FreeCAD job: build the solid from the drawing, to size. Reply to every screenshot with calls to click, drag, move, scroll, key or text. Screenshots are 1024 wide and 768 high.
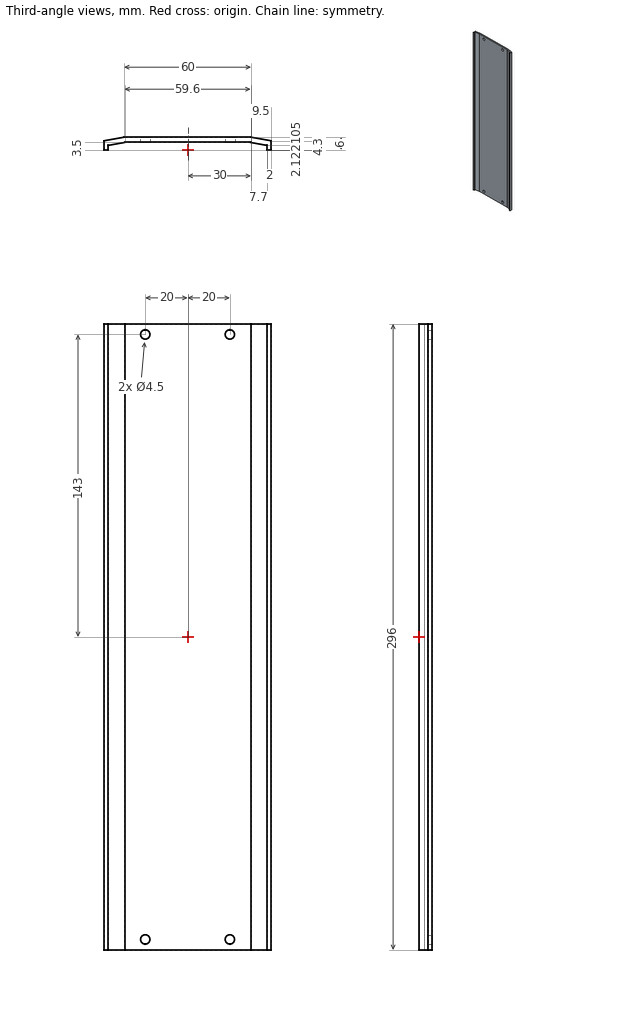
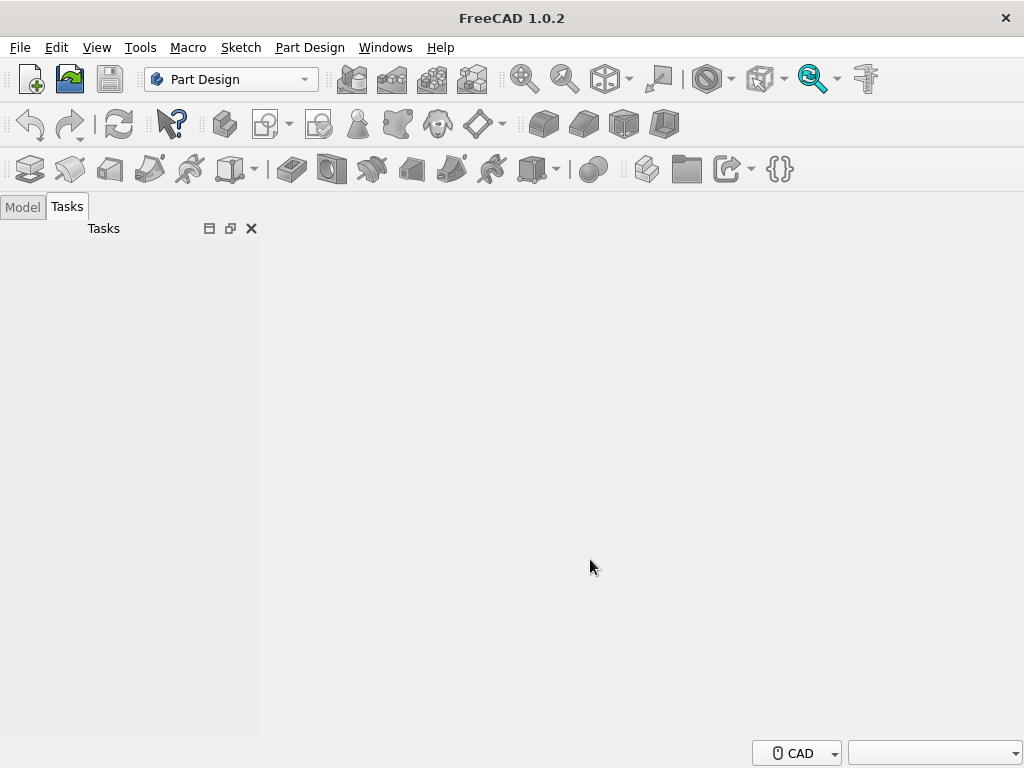
key(ctrl+n)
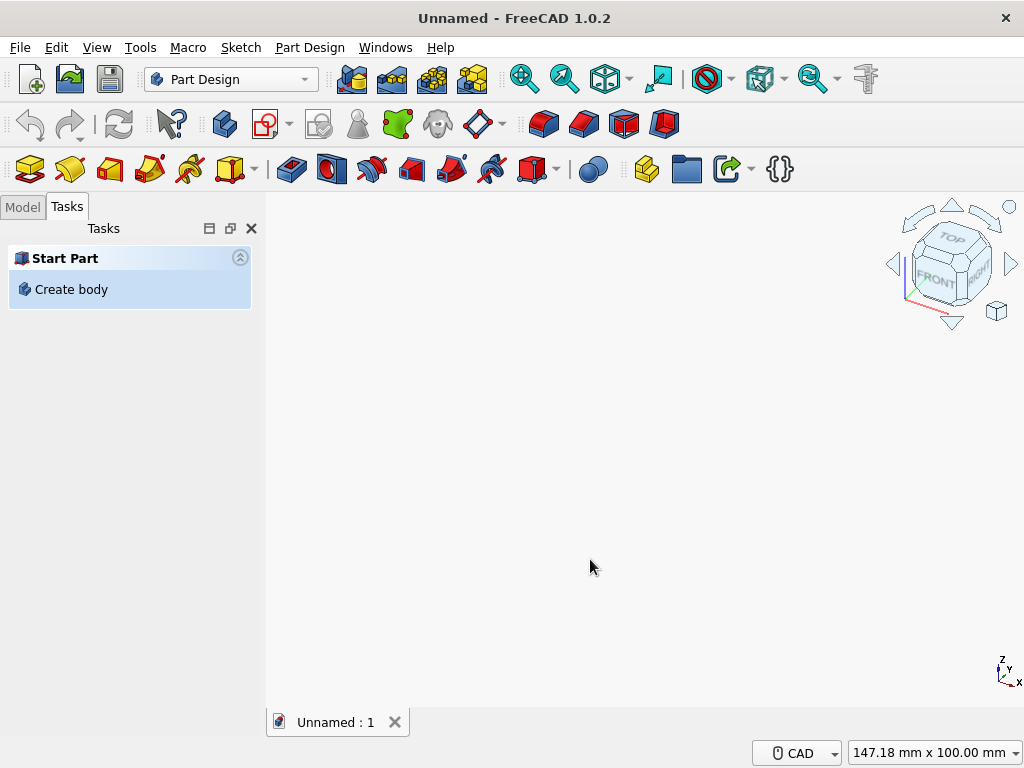
click(266, 124)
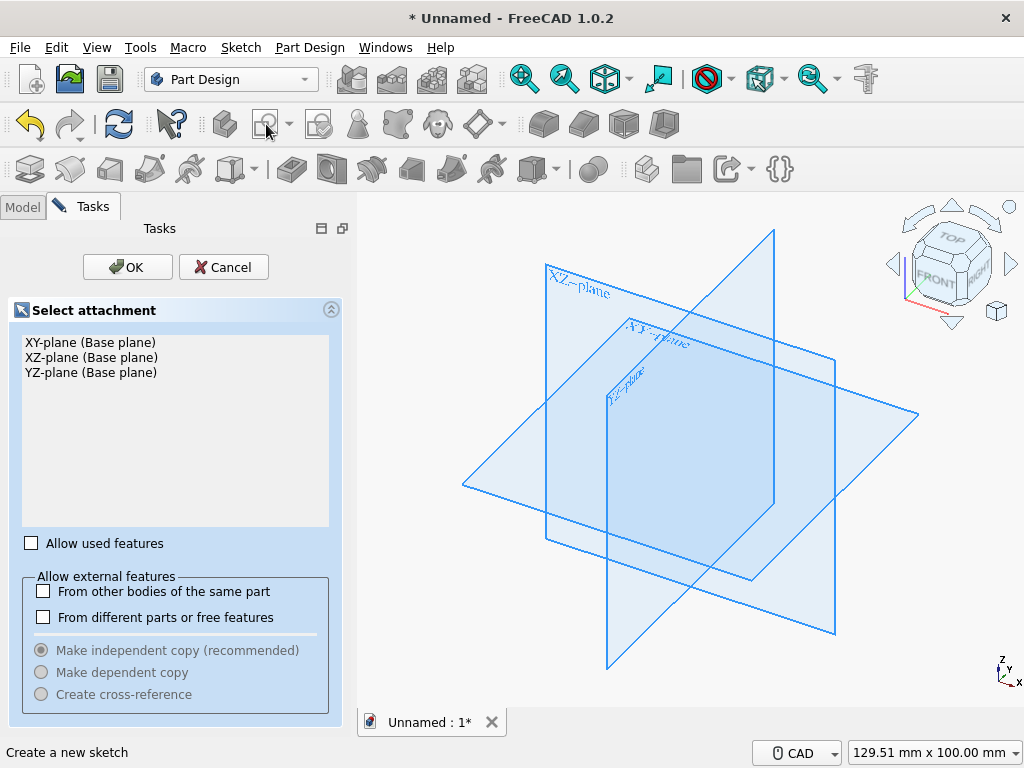
click(82, 342)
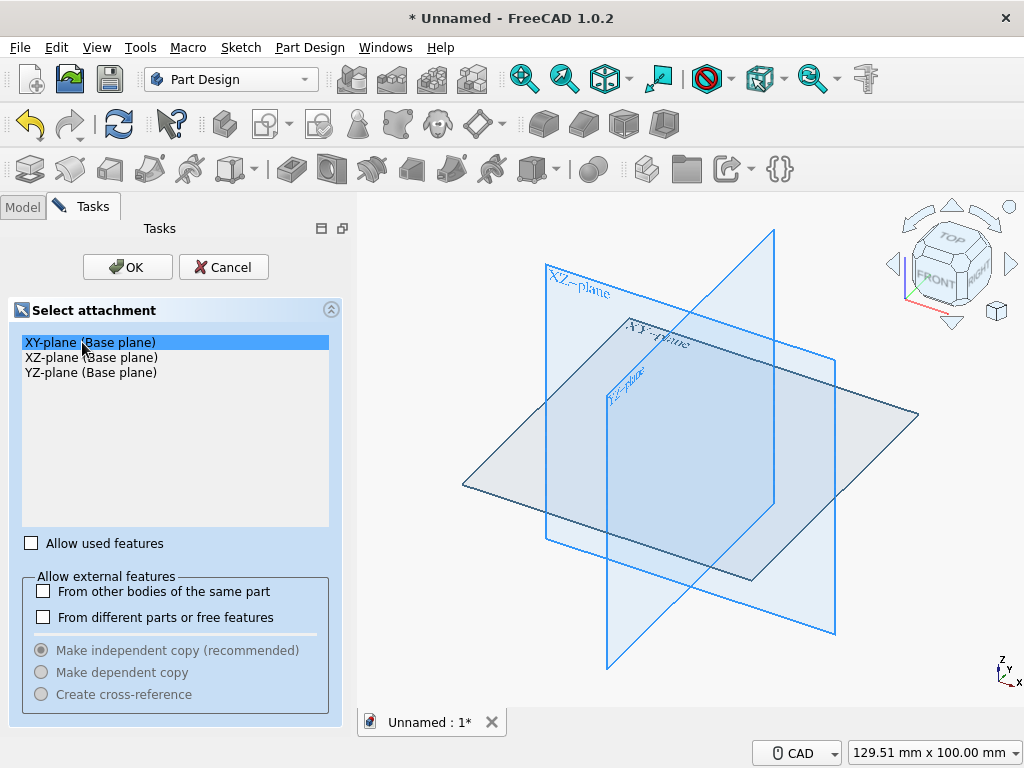
click(128, 267)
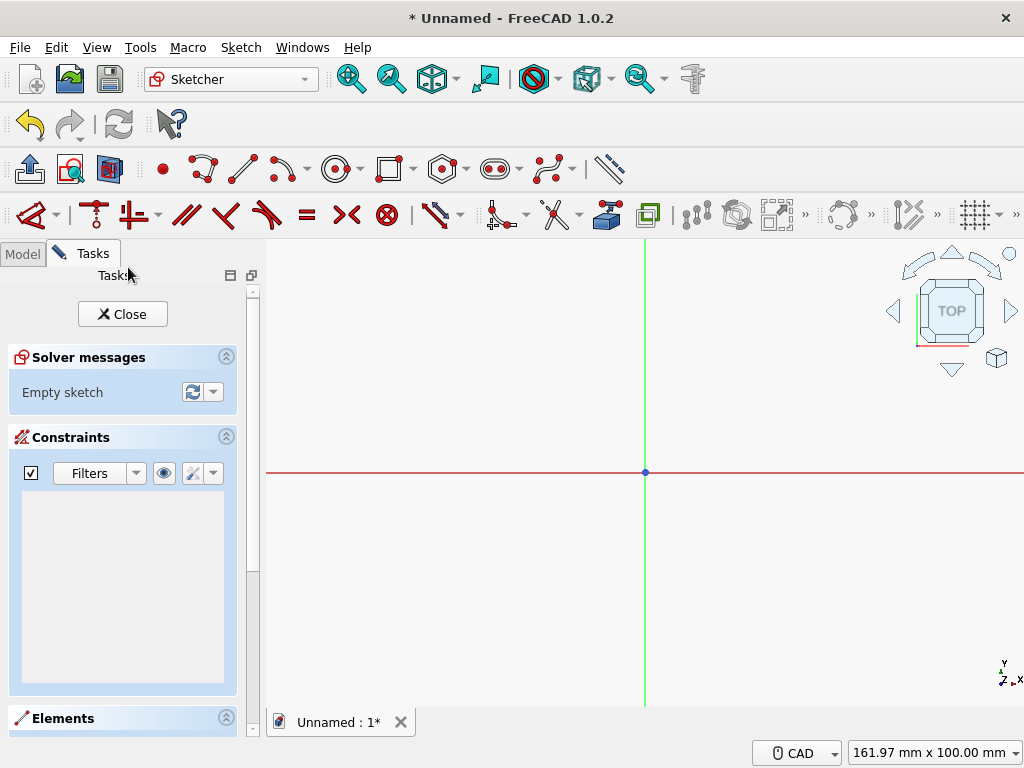
key(g)
key(m)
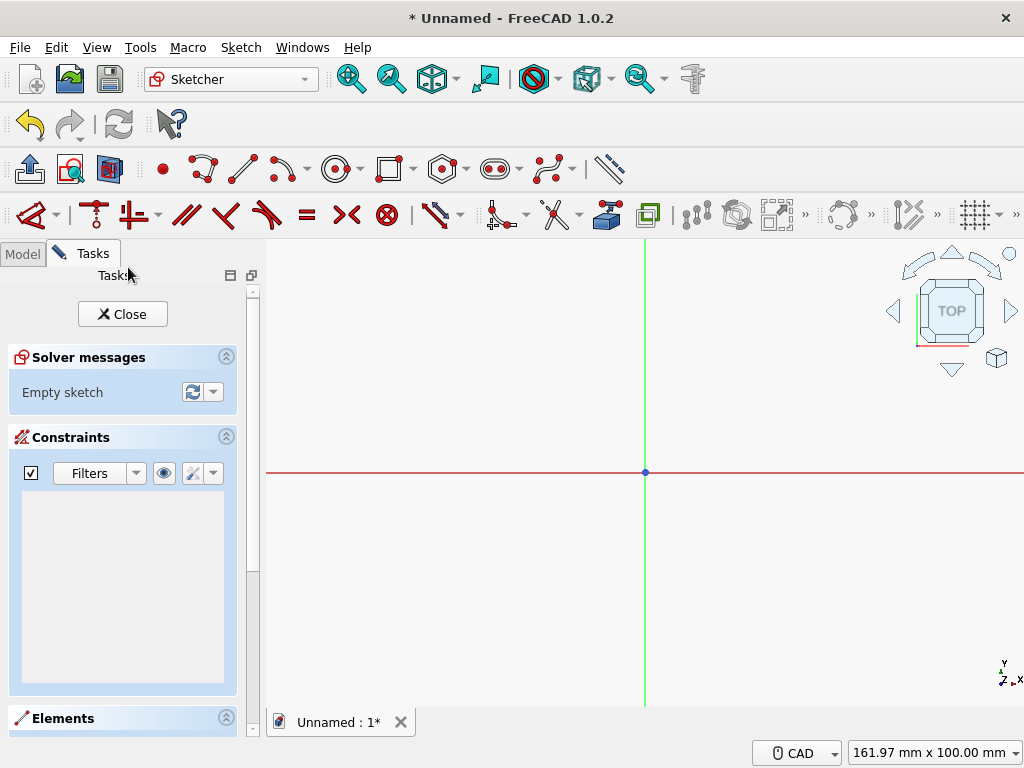
click(506, 457)
click(784, 457)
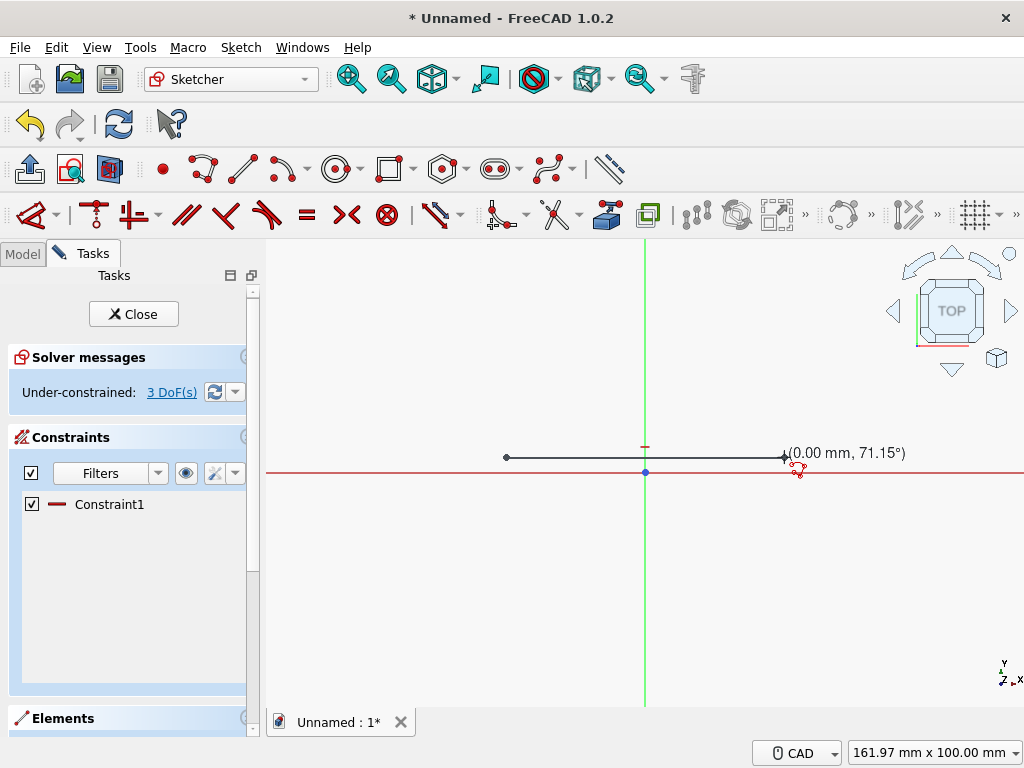
scroll(820, 463, up, 3)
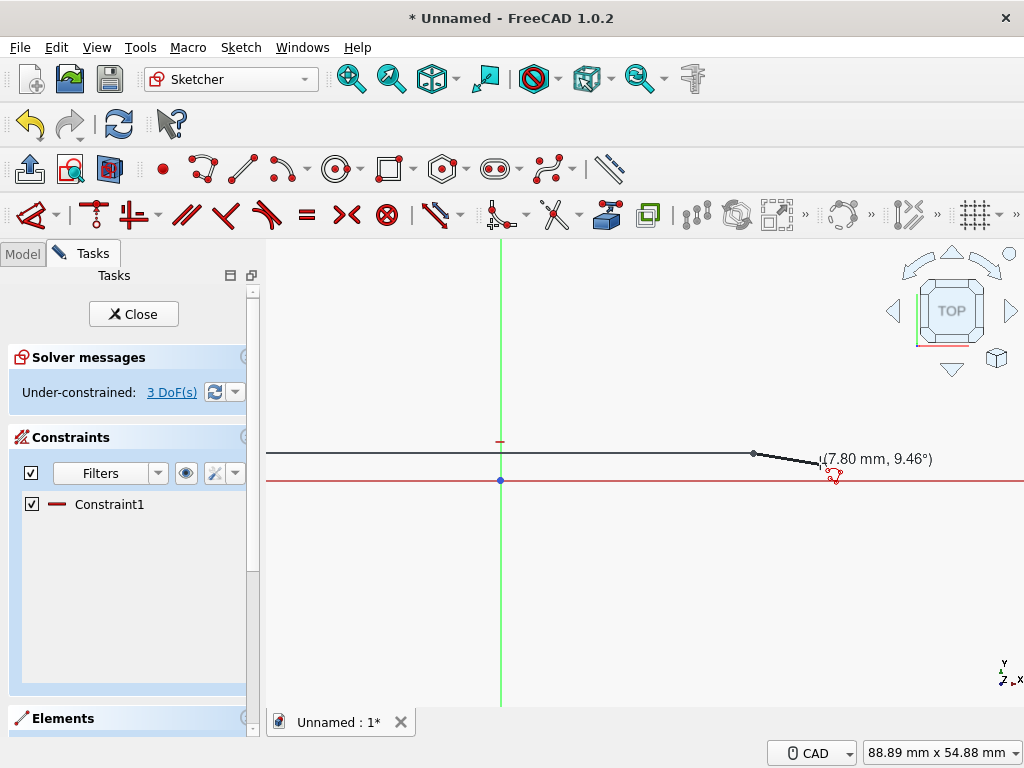
click(820, 463)
click(820, 481)
click(837, 472)
click(837, 444)
click(756, 430)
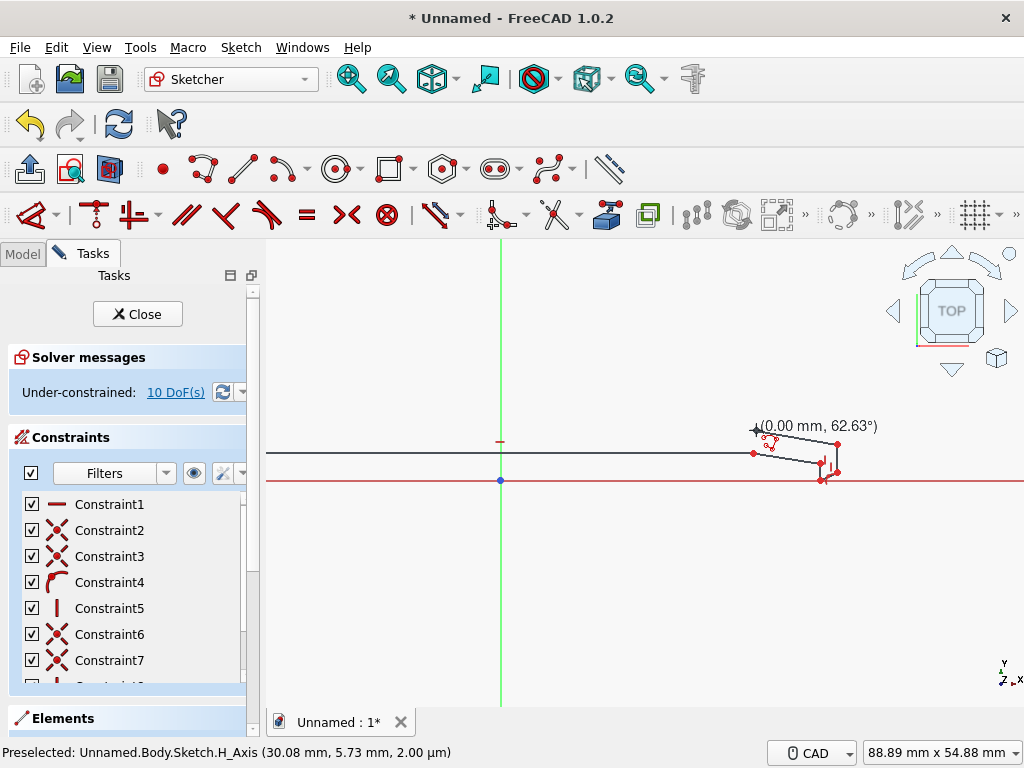
scroll(669, 495, down, 3)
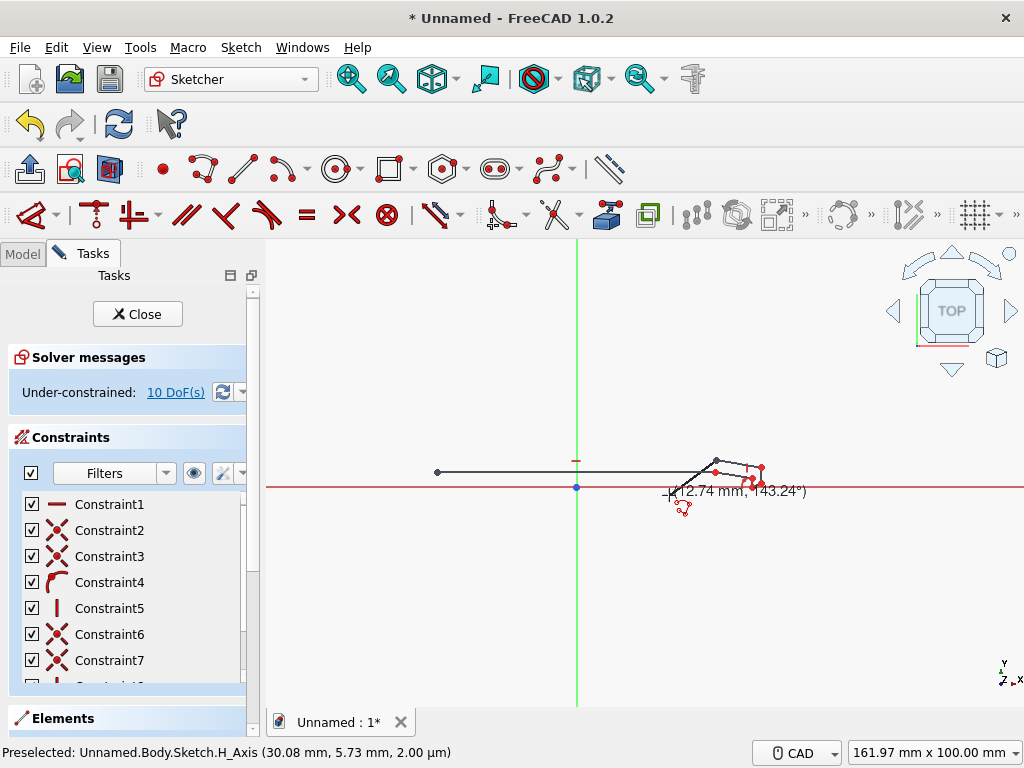
scroll(436, 459, up, 2)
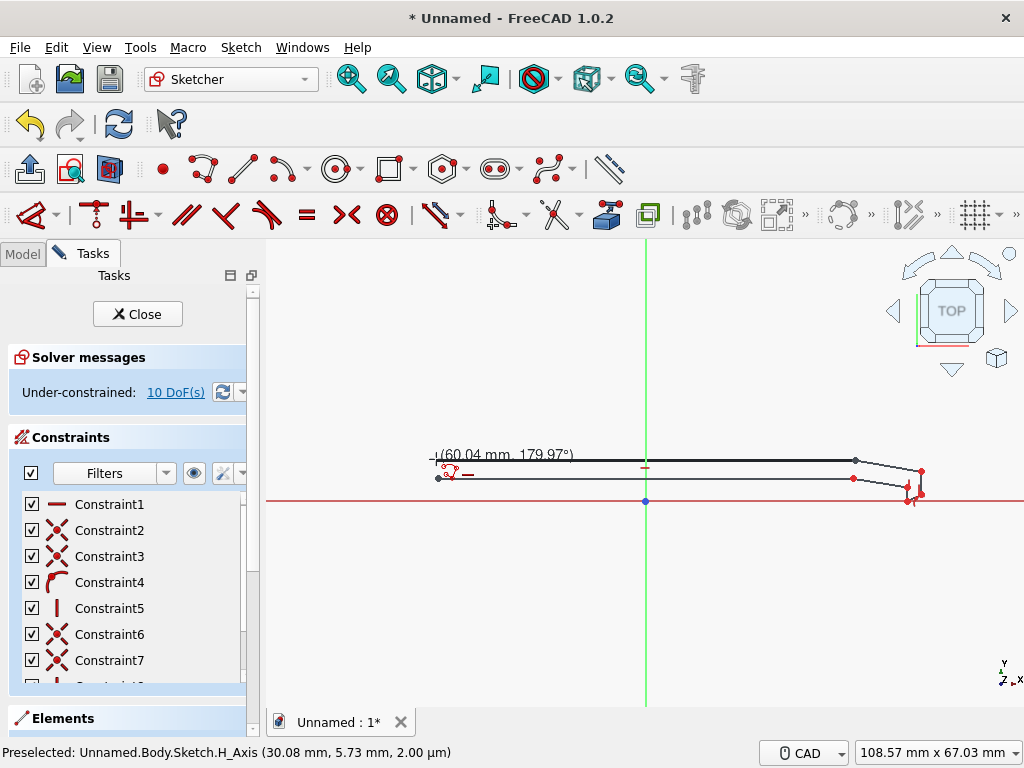
click(436, 460)
click(370, 471)
click(370, 501)
click(384, 492)
click(384, 486)
click(439, 479)
key(Escape)
key(Escape)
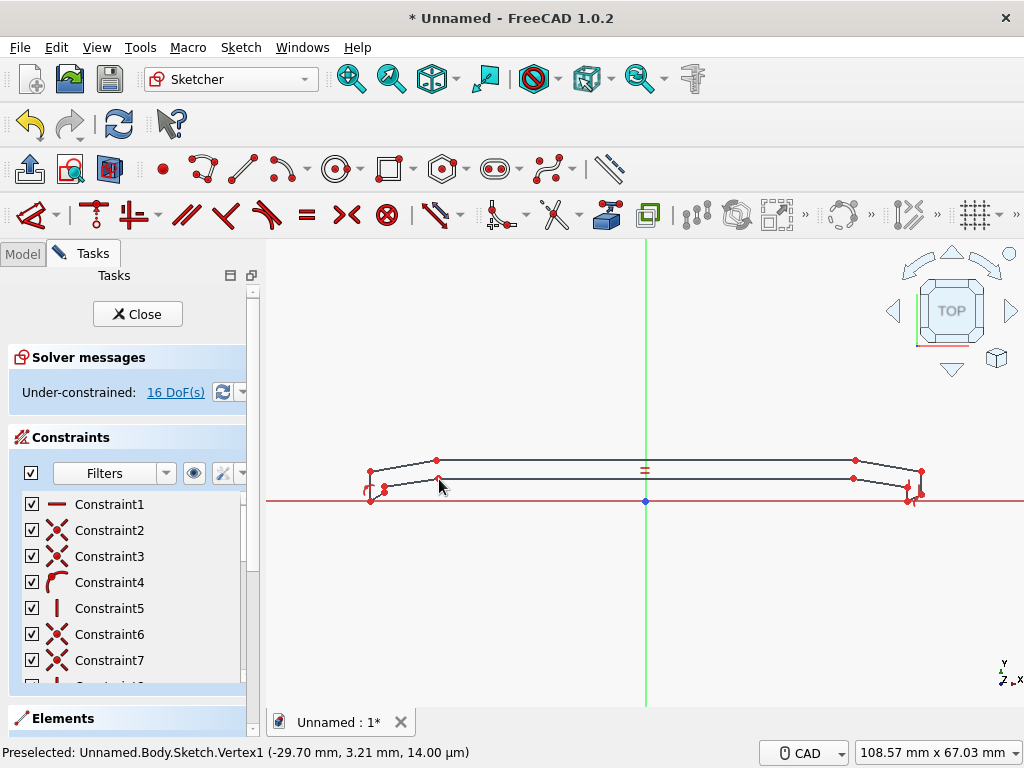
scroll(435, 458, down, 2)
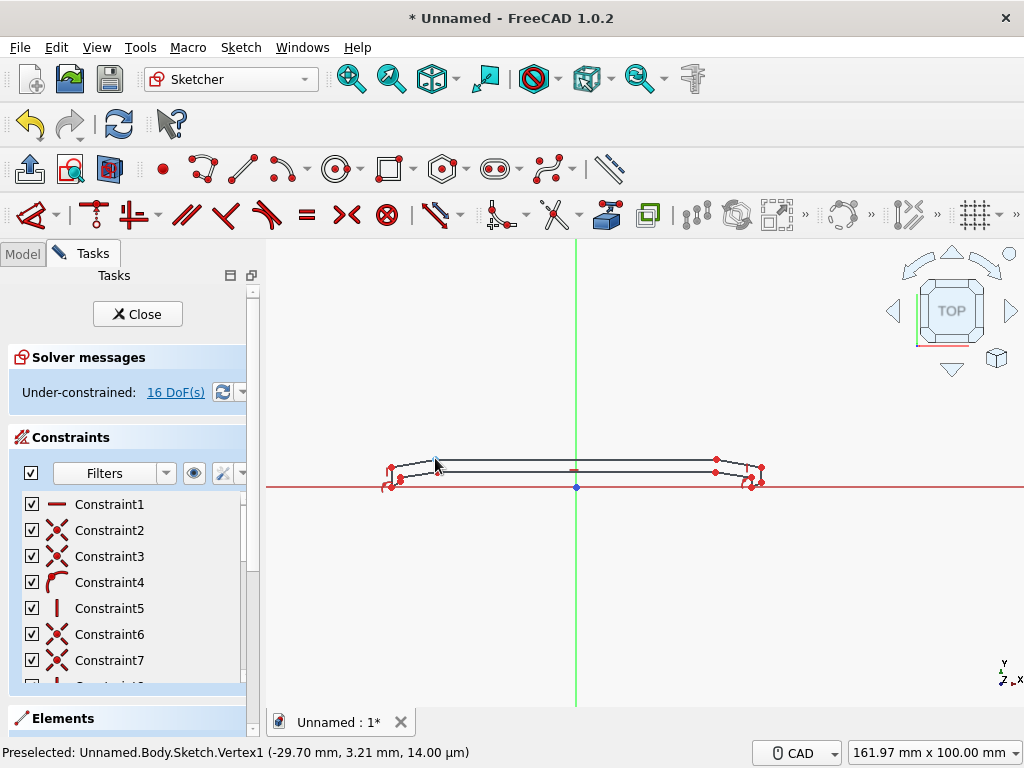
scroll(756, 485, up, 6)